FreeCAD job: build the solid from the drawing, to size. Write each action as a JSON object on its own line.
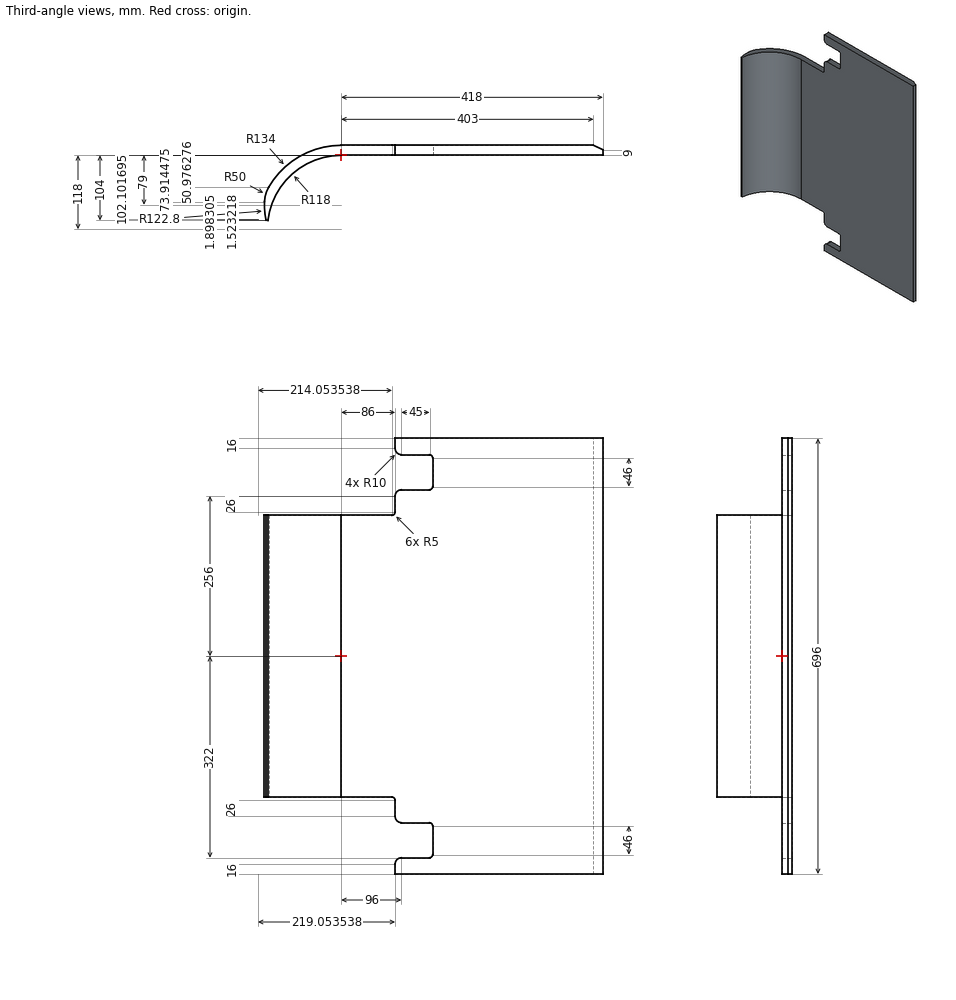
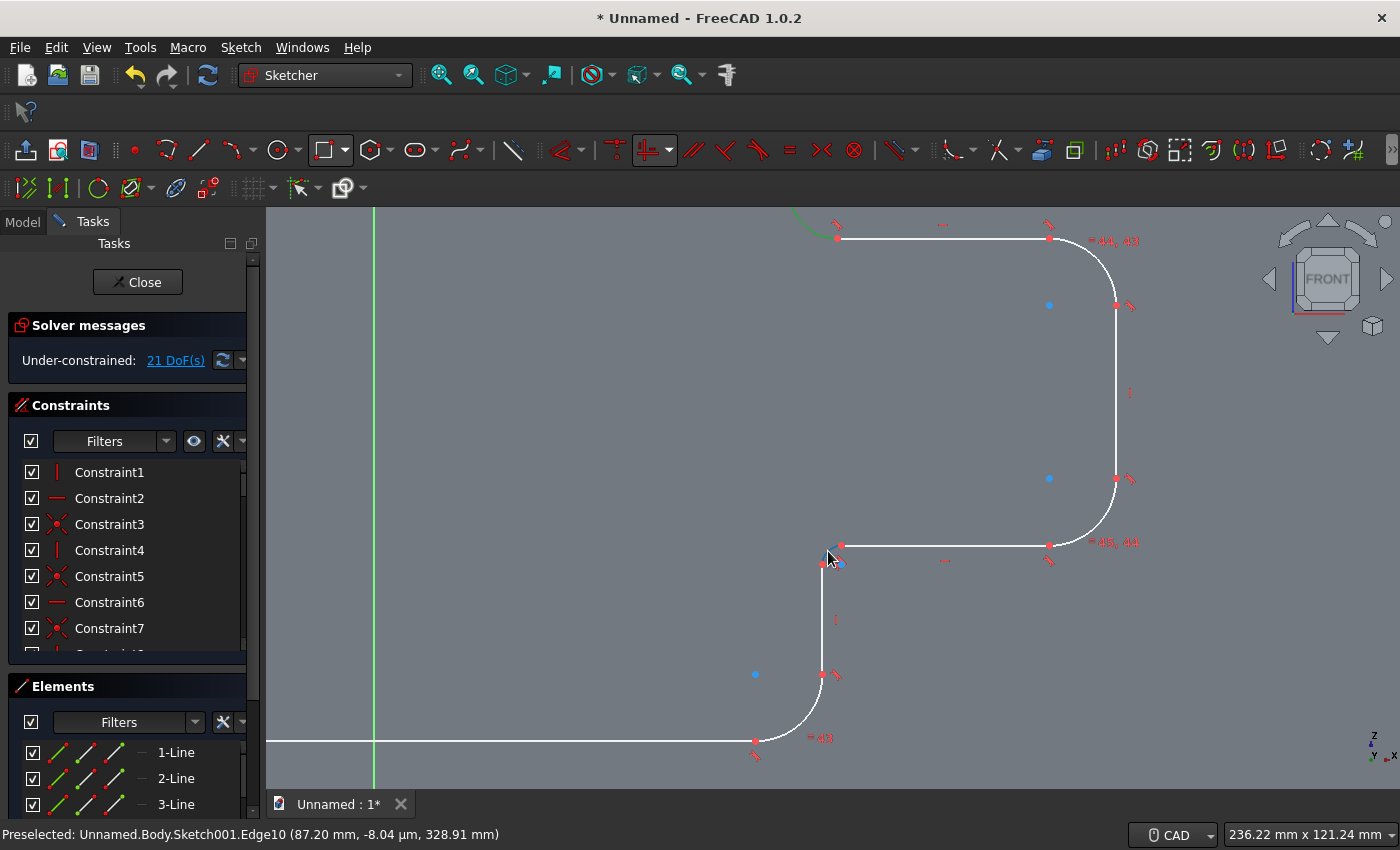
{"action": "left_click", "coordinate": [828, 551]}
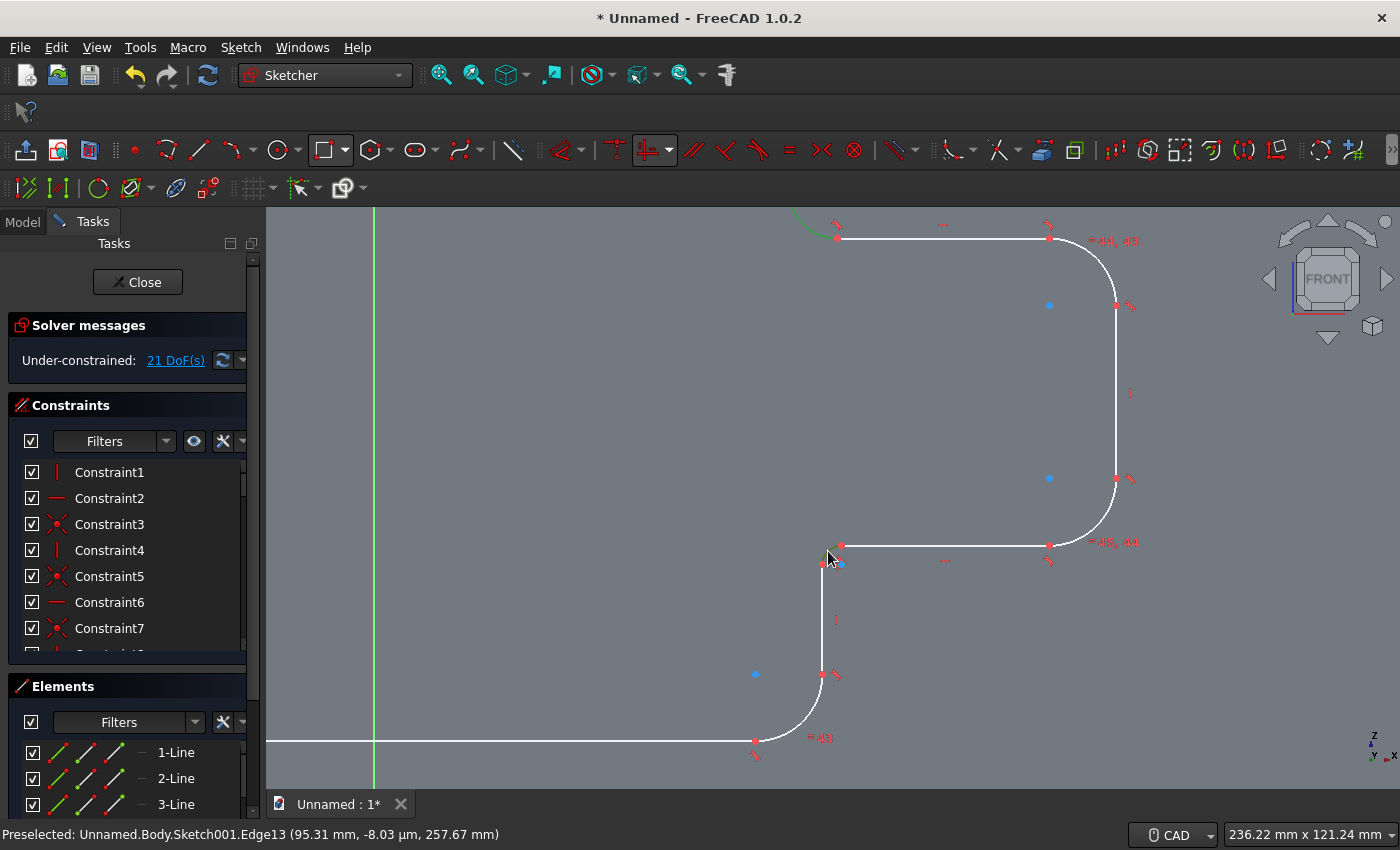
{"action": "scroll", "coordinate": [809, 338], "scroll_direction": "down", "scroll_amount": 11}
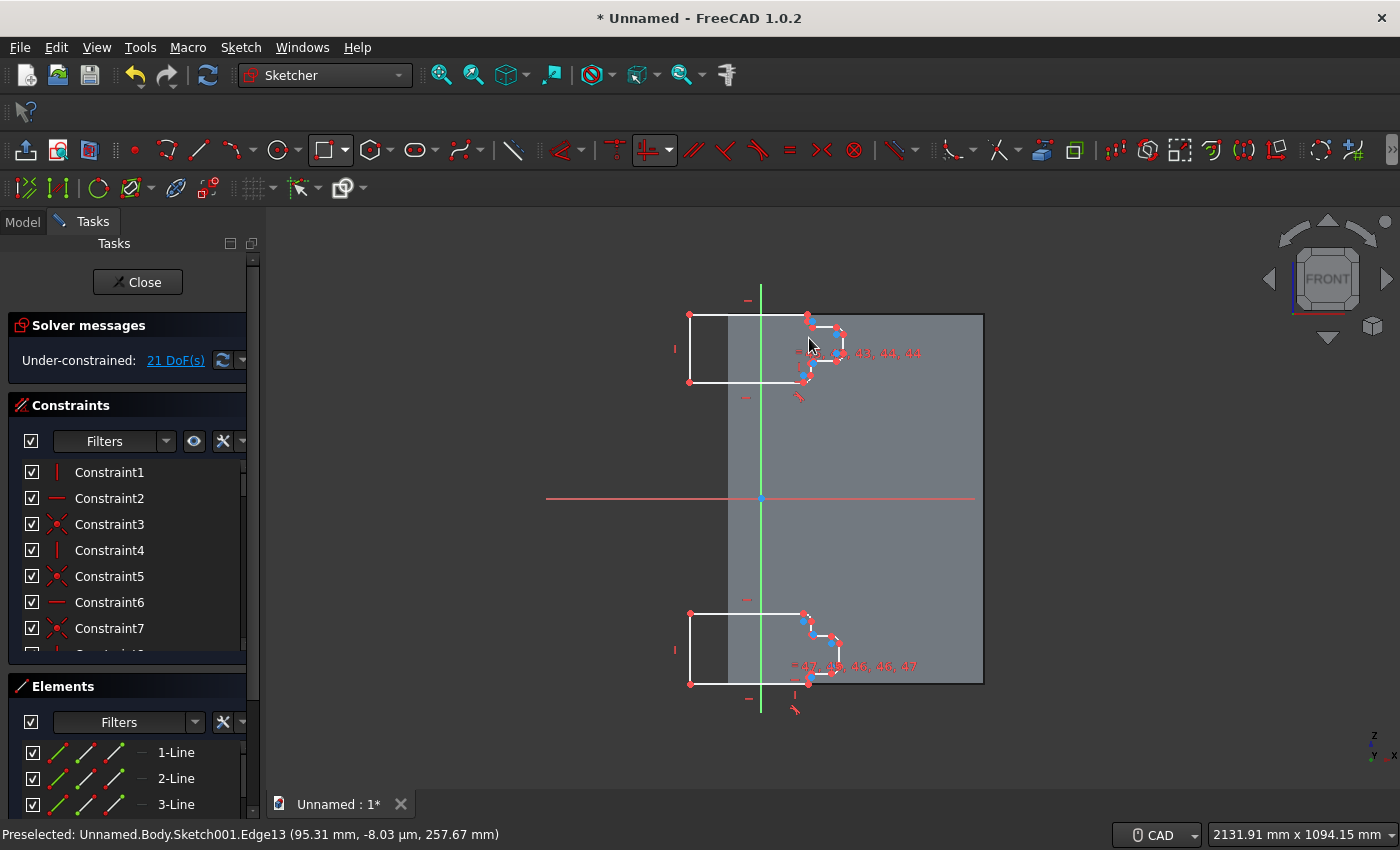
{"action": "scroll", "coordinate": [810, 674], "scroll_direction": "up", "scroll_amount": 12}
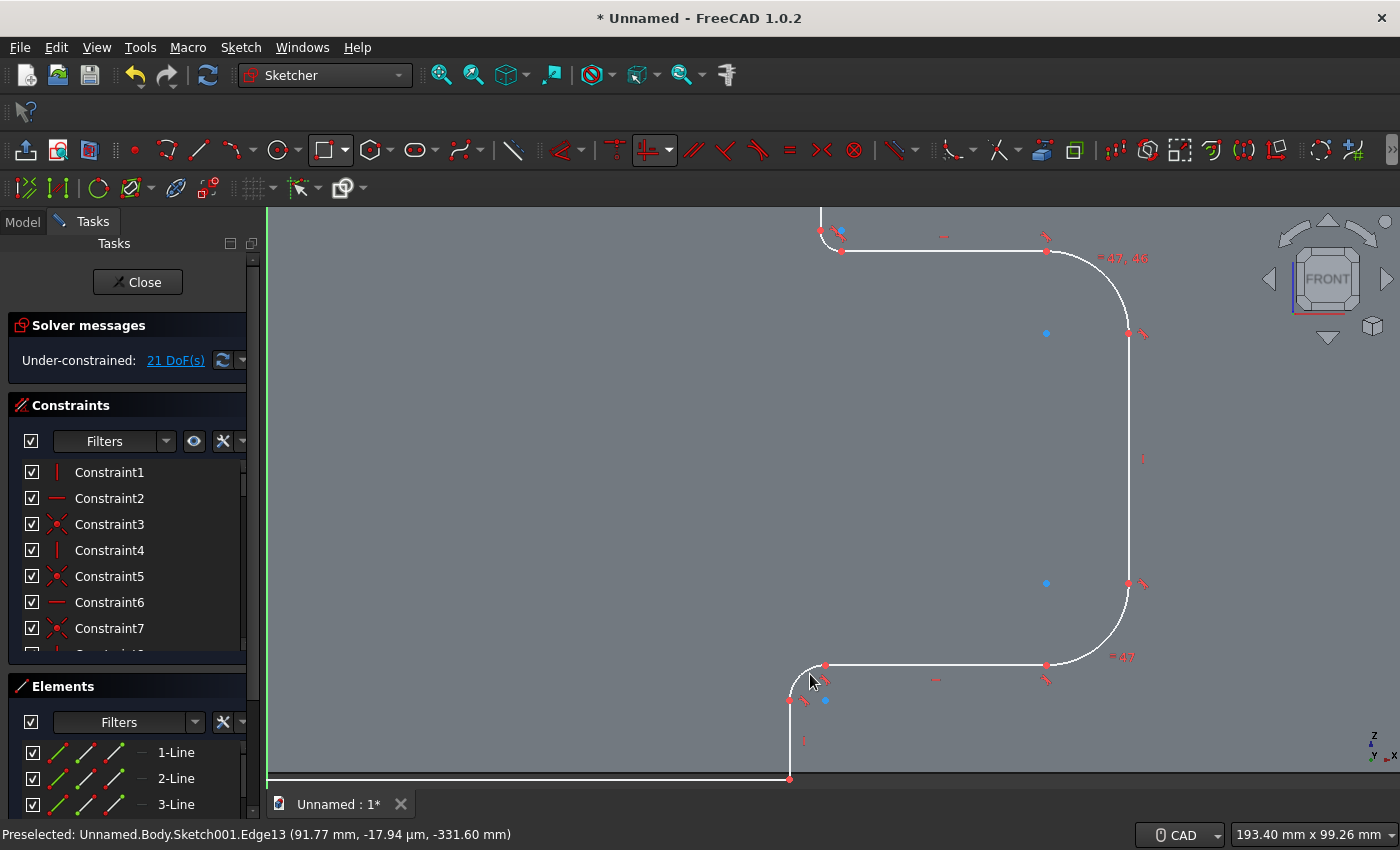
{"action": "left_click", "coordinate": [809, 669]}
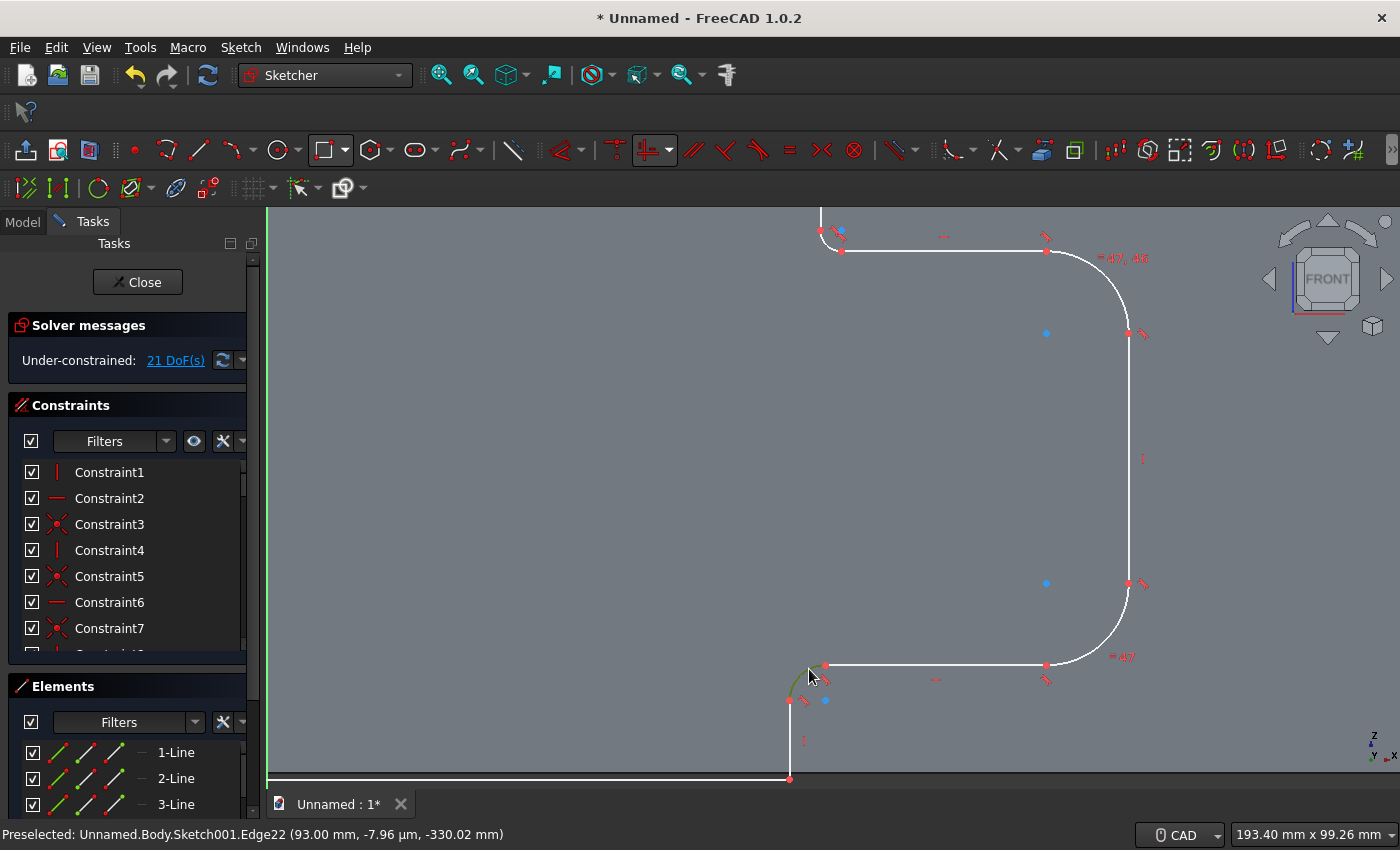
{"action": "scroll", "coordinate": [823, 240], "scroll_direction": "up", "scroll_amount": 2}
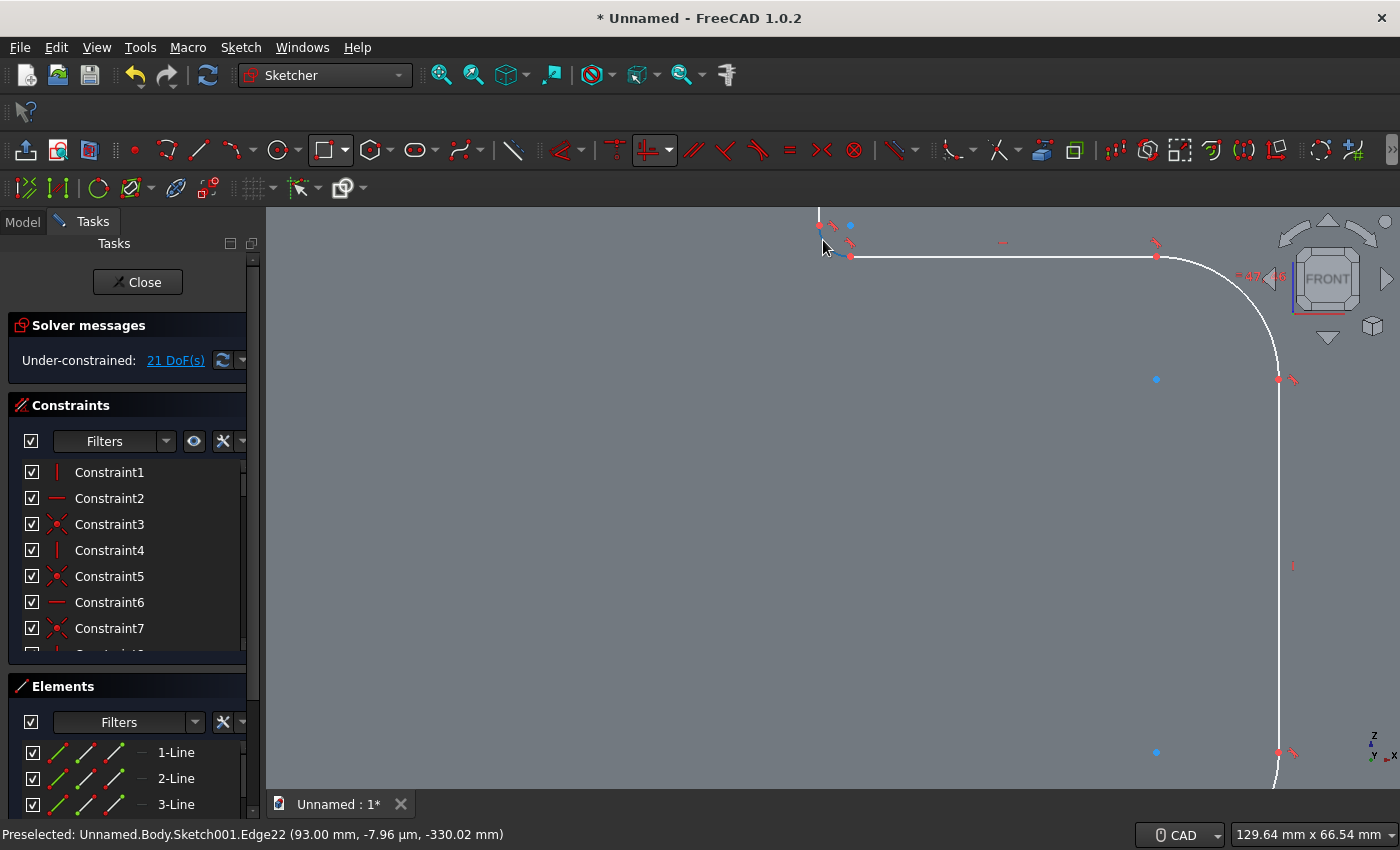
{"action": "left_click", "coordinate": [823, 240]}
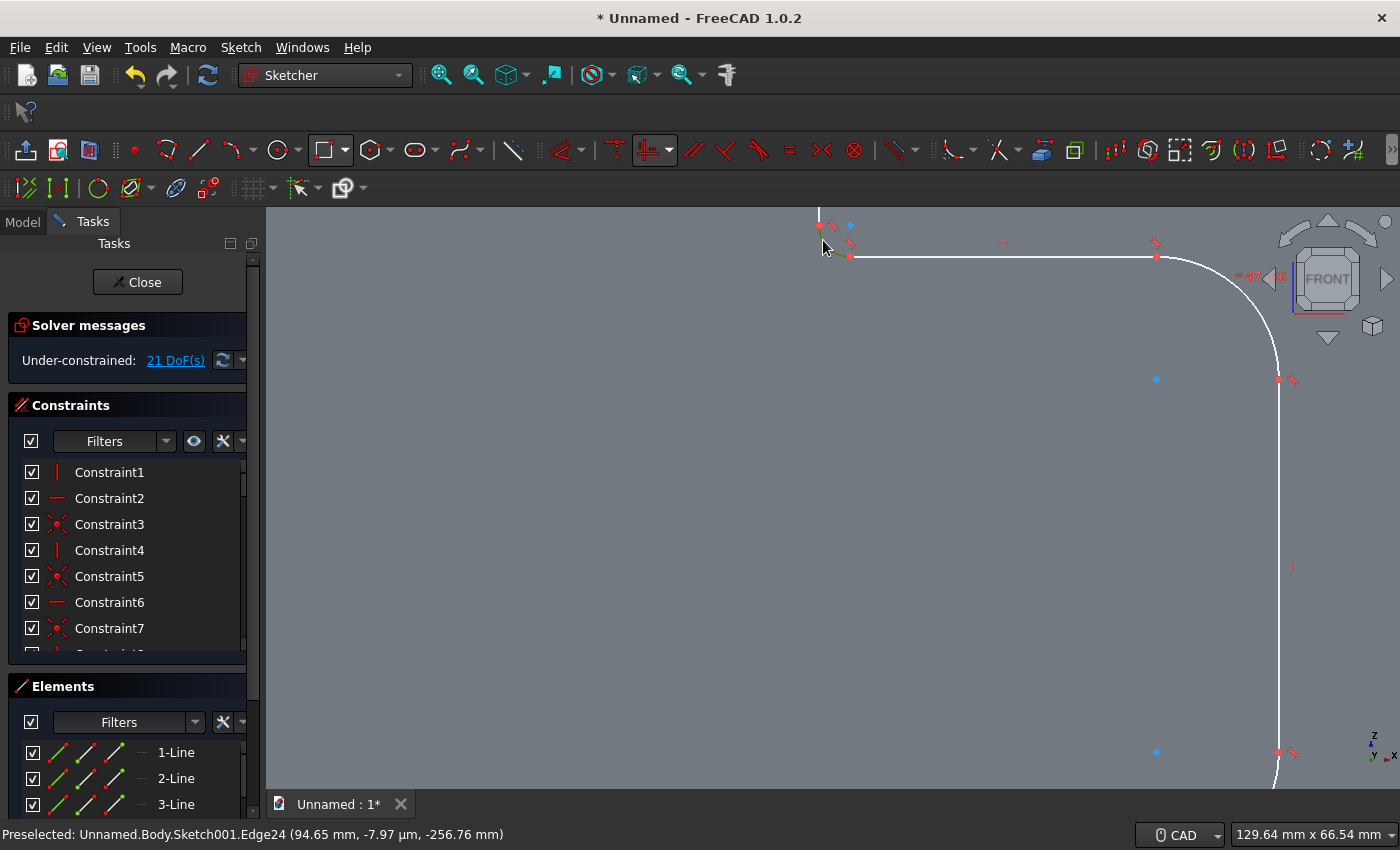
{"action": "left_click", "coordinate": [790, 150]}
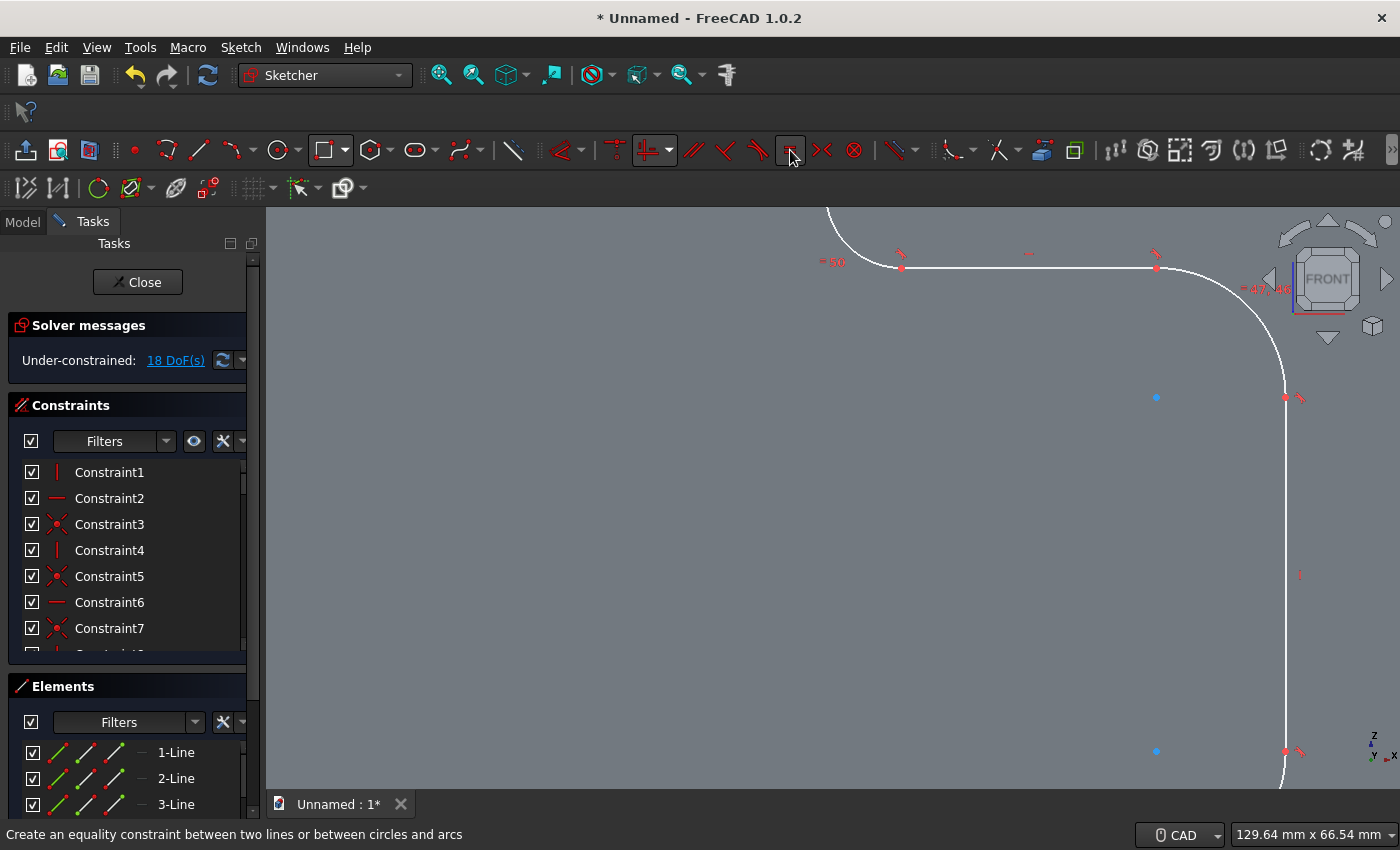
{"action": "left_click", "coordinate": [560, 150]}